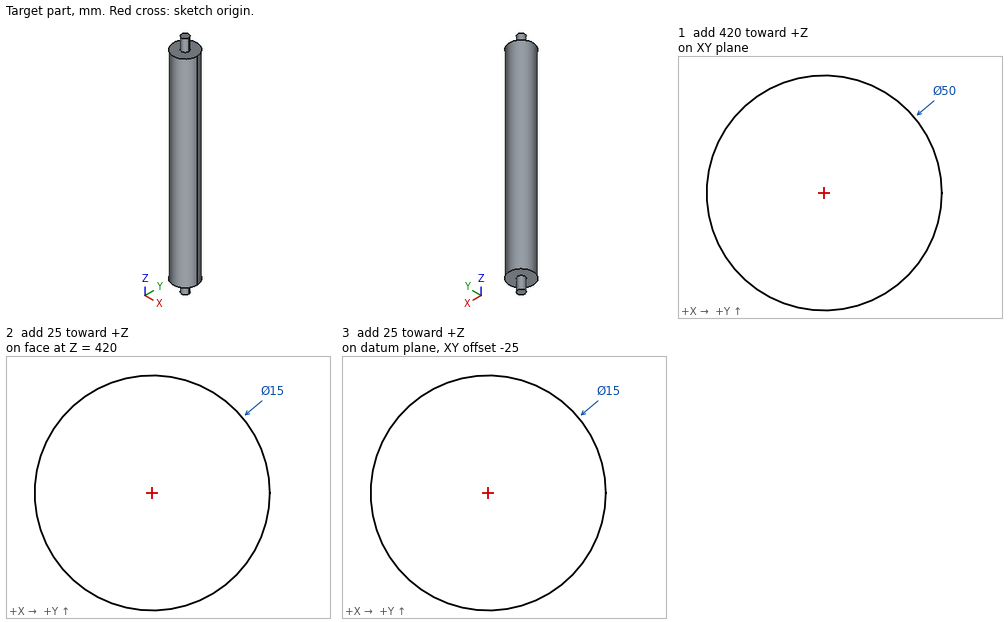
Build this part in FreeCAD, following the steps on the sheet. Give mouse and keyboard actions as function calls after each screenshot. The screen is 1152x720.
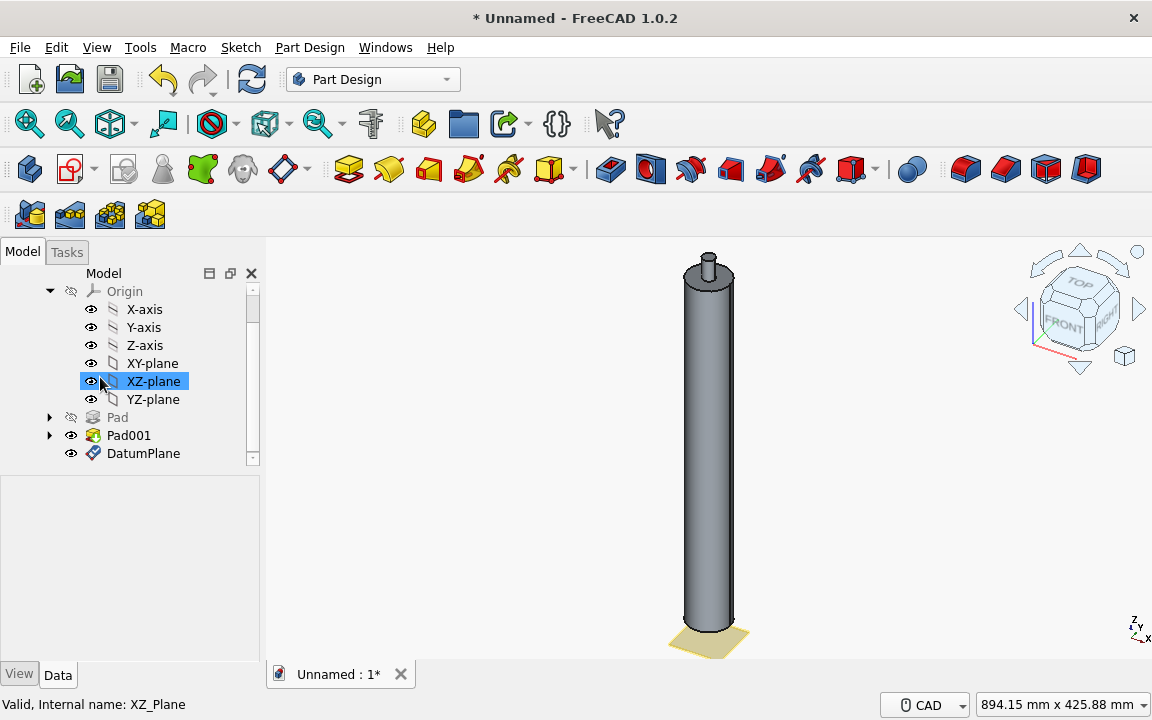
click(116, 453)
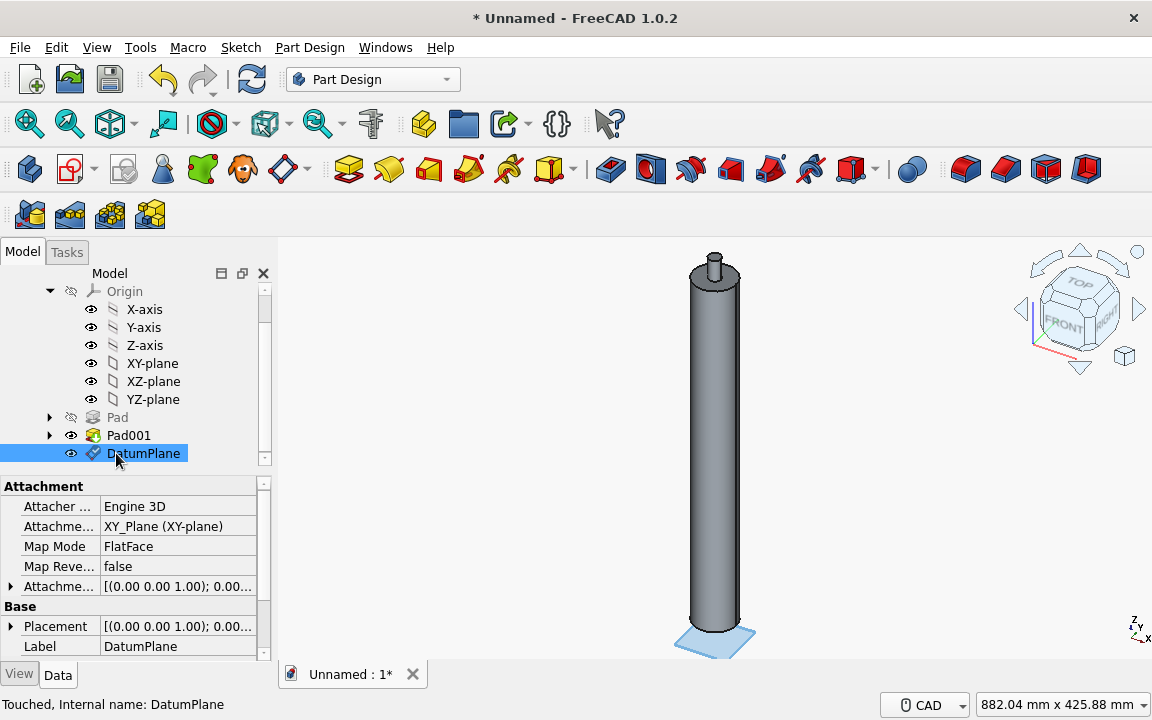
click(70, 170)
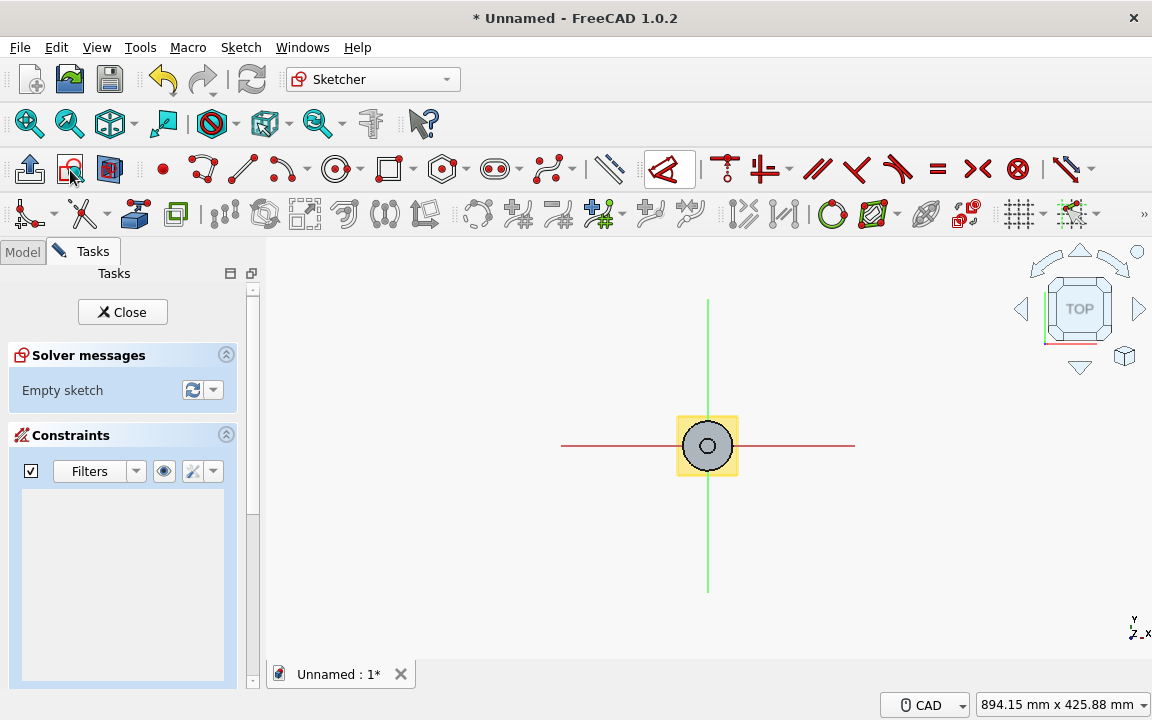
key(q)
key(s)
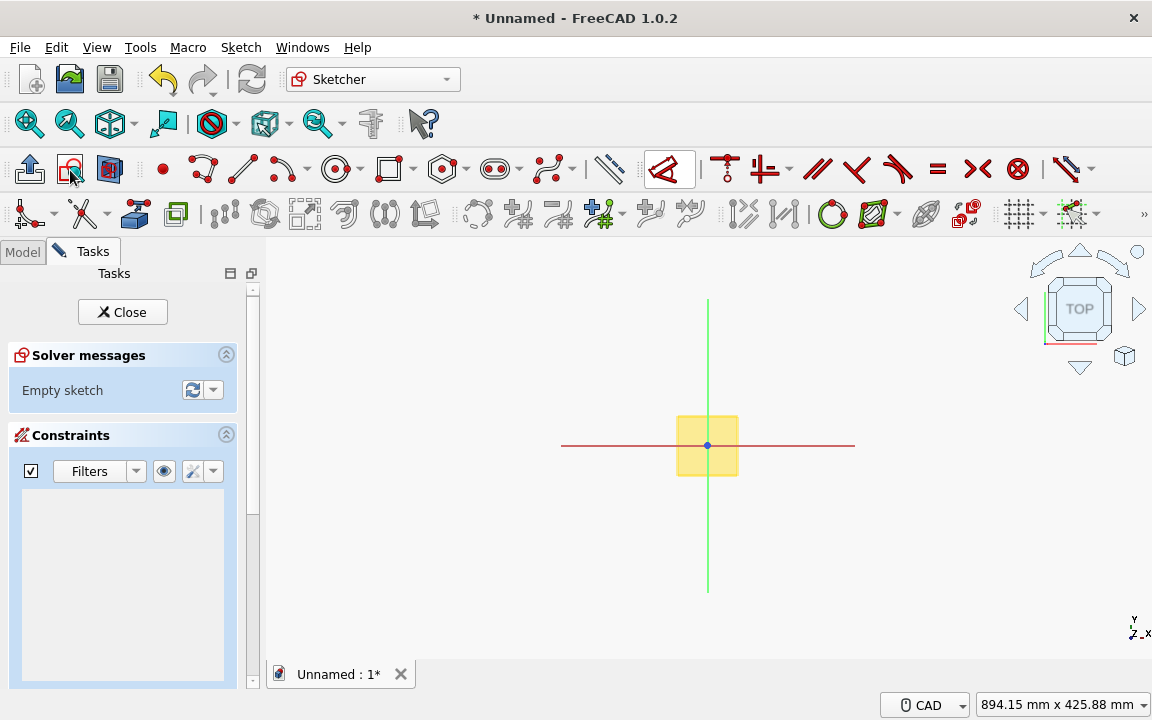
scroll(712, 446, up, 14)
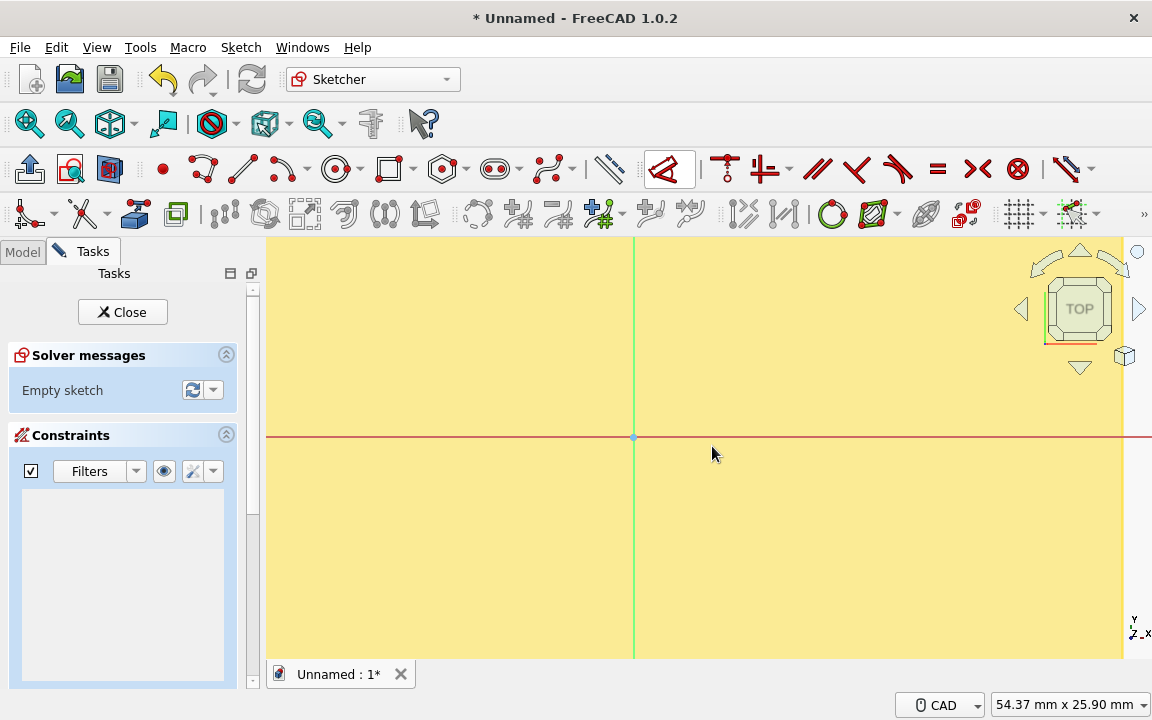
key(g)
key(c)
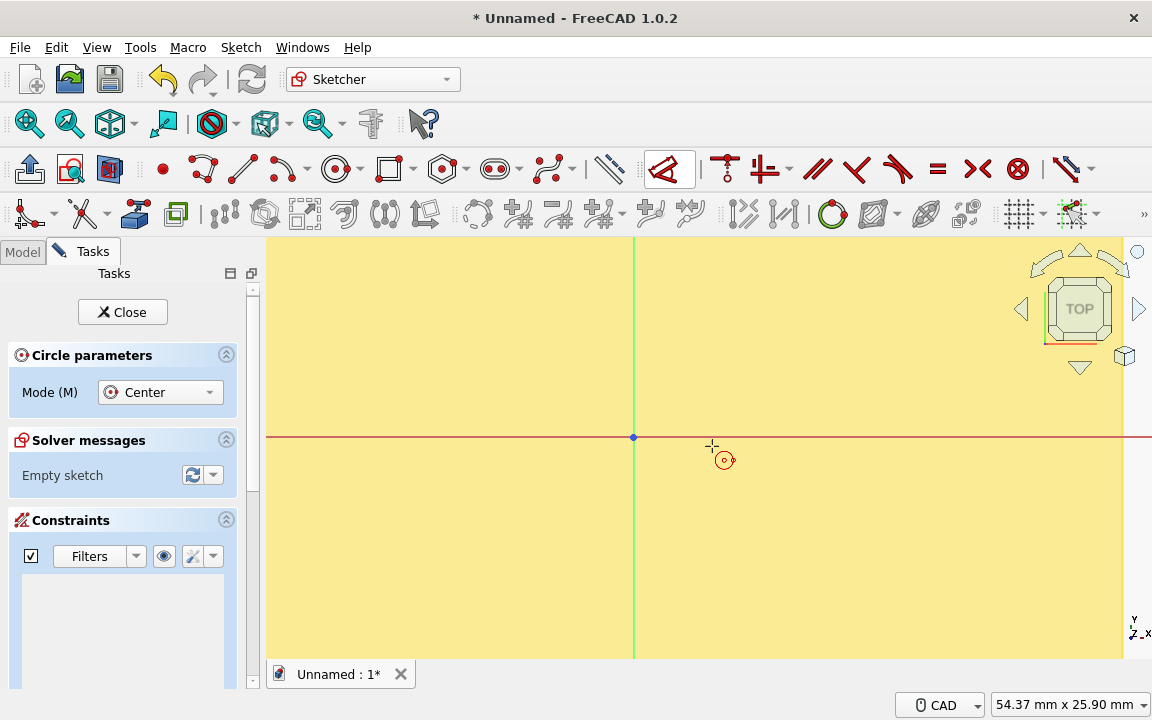
click(634, 437)
click(720, 351)
key(Escape)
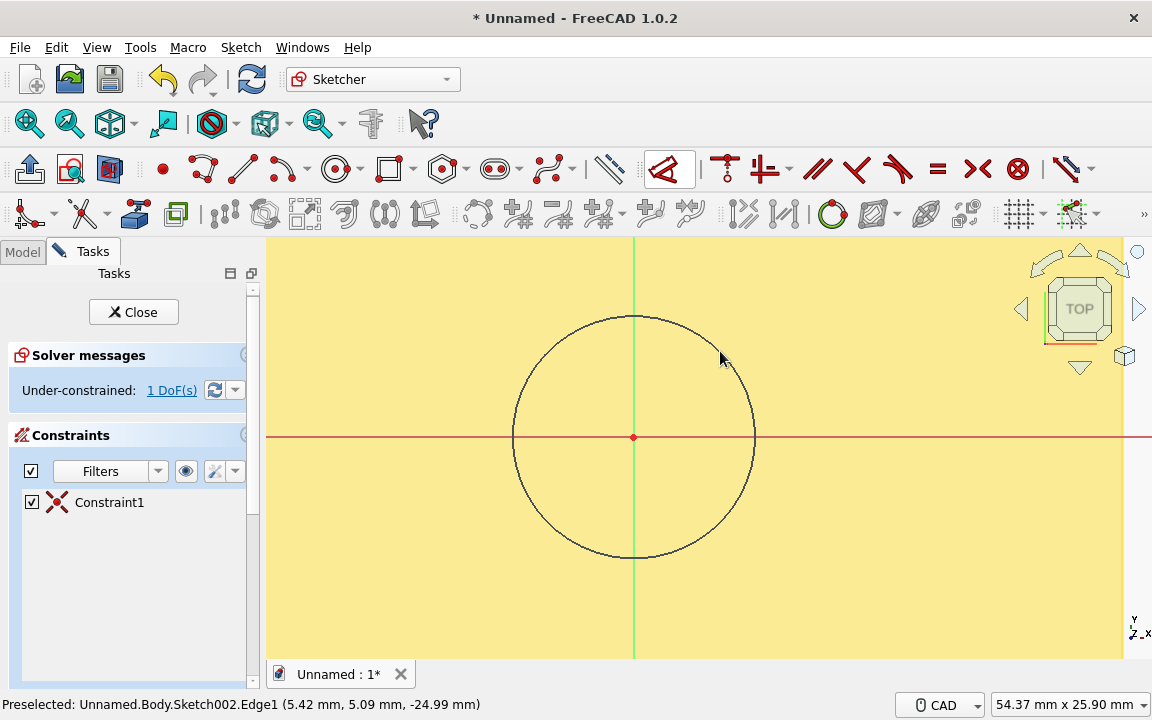
key(d)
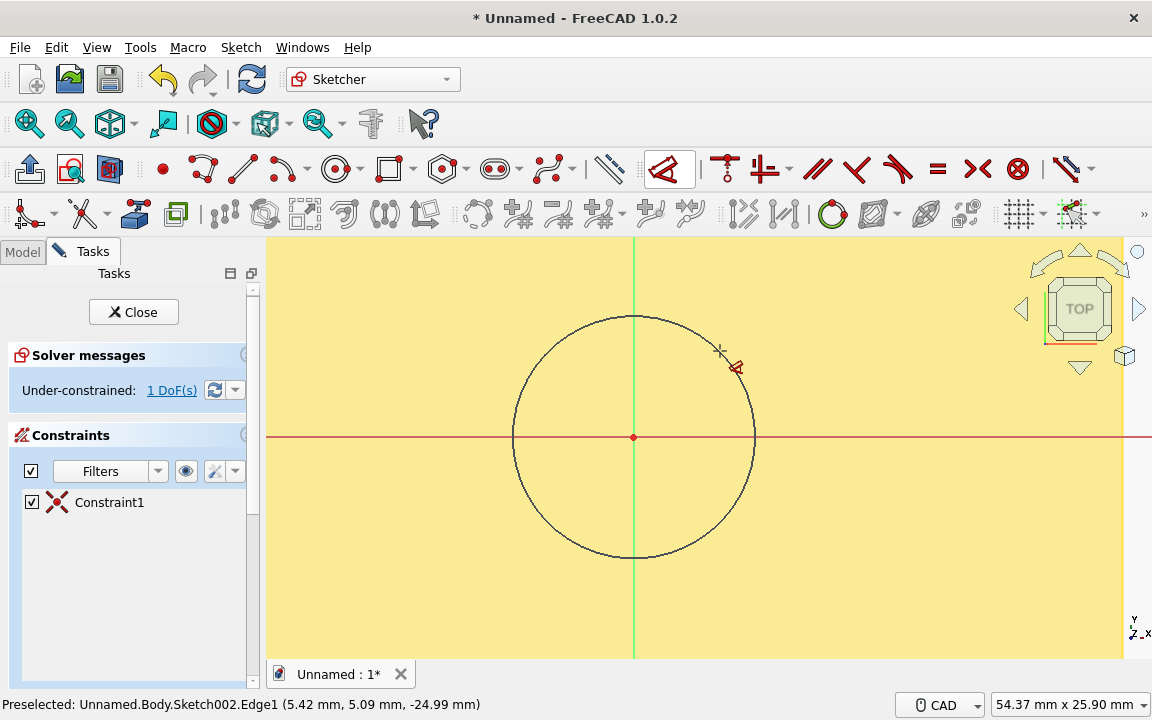
click(719, 351)
click(741, 328)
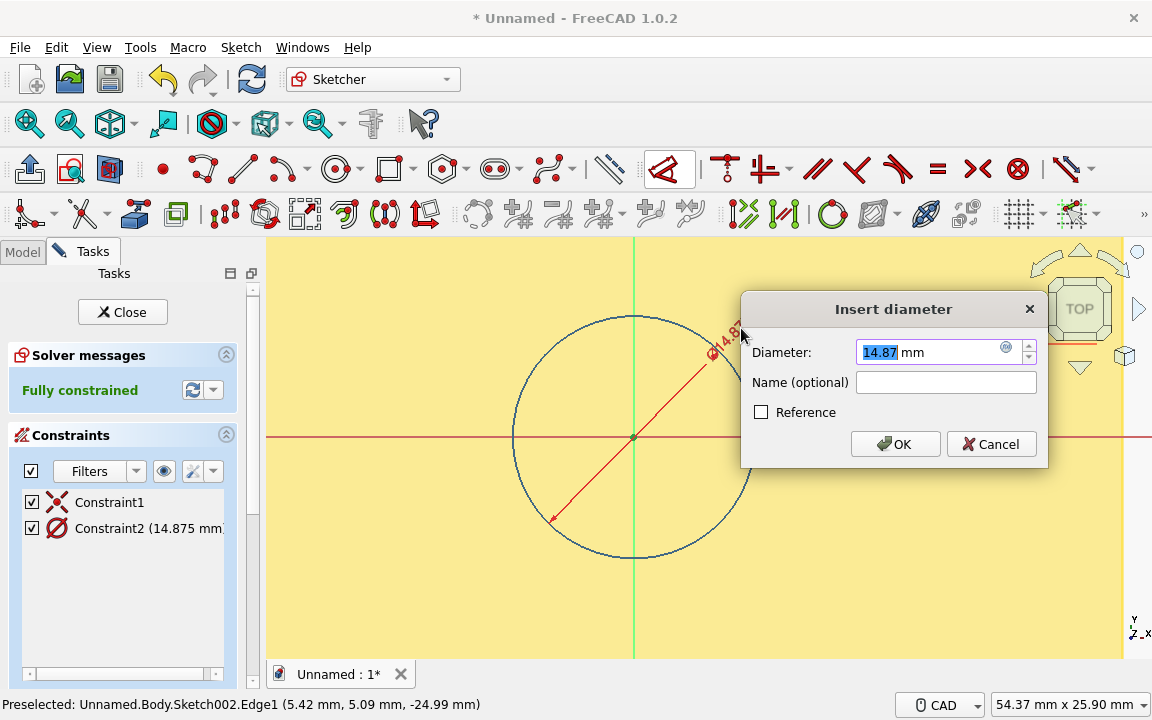
text(15)
key(Return)
key(Escape)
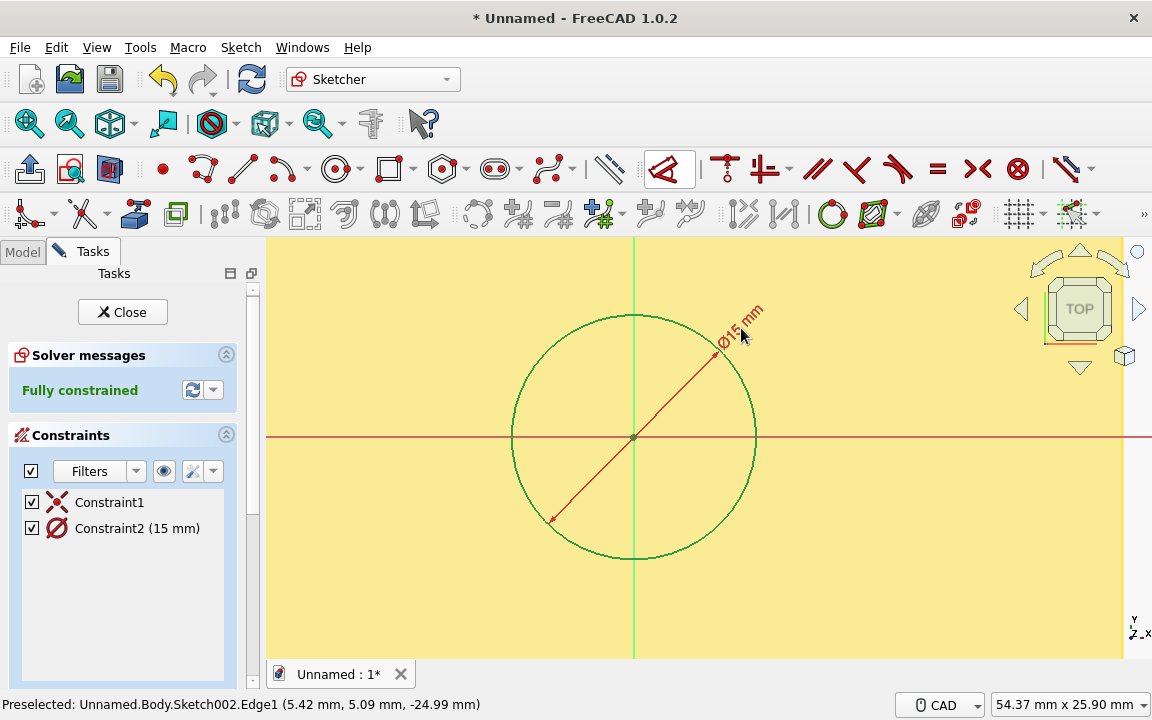
click(123, 312)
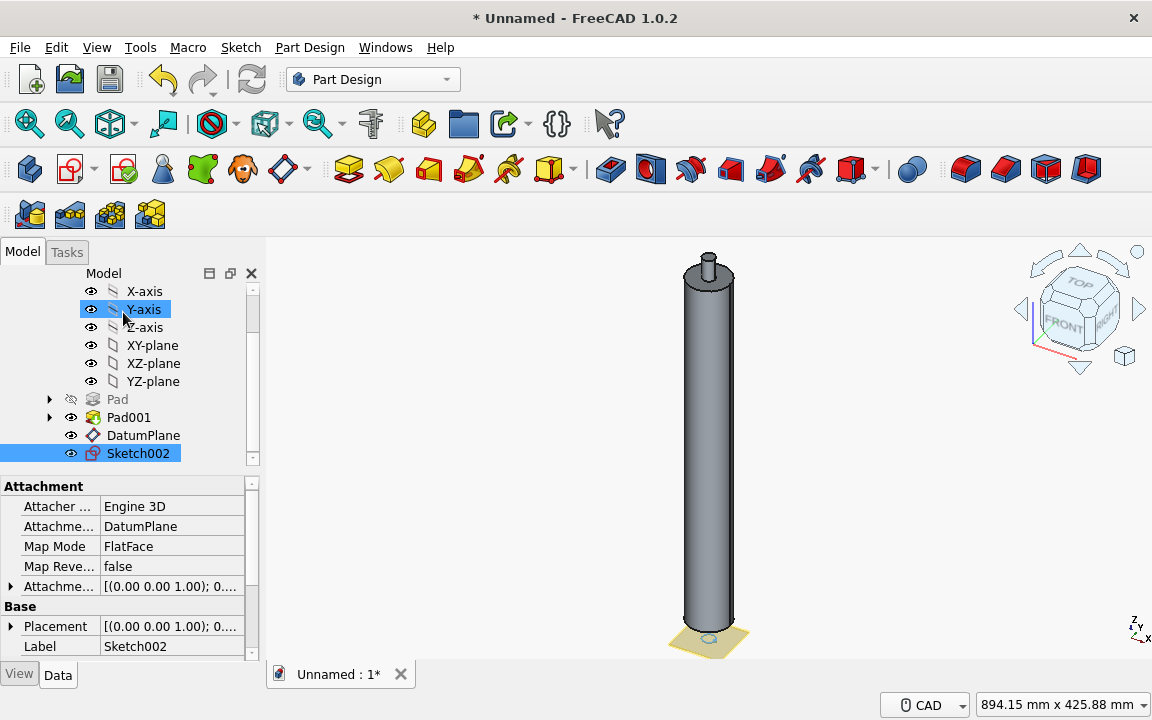
click(350, 170)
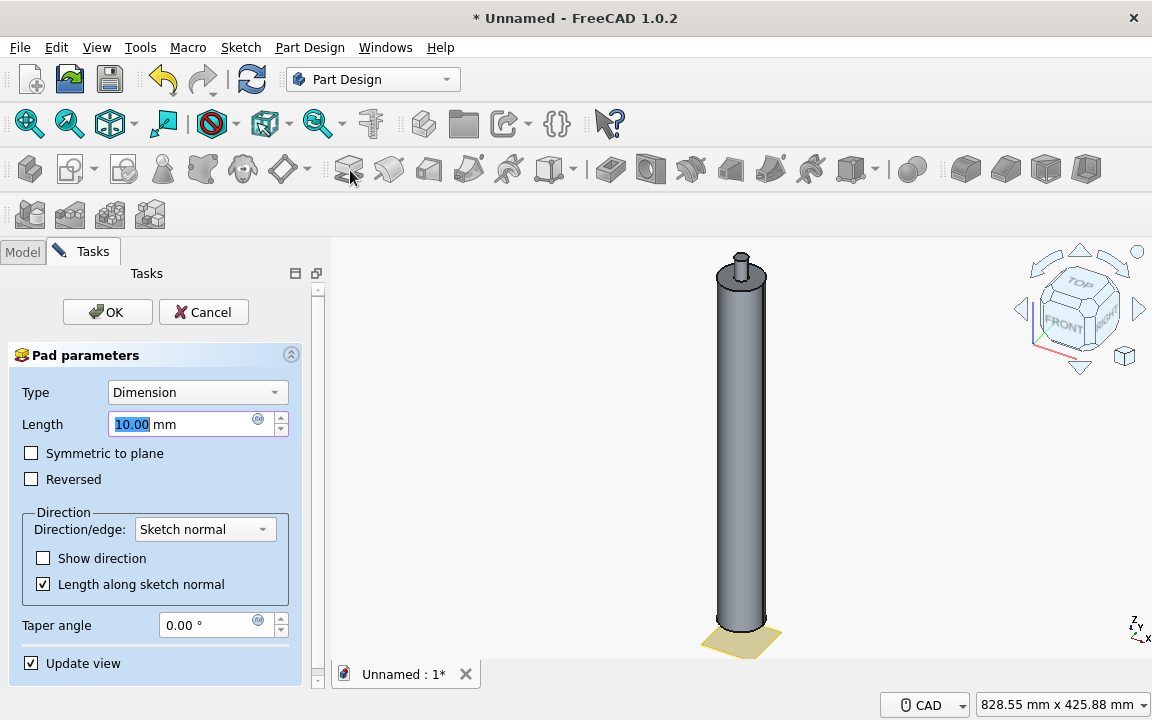
text(25)
key(Tab)